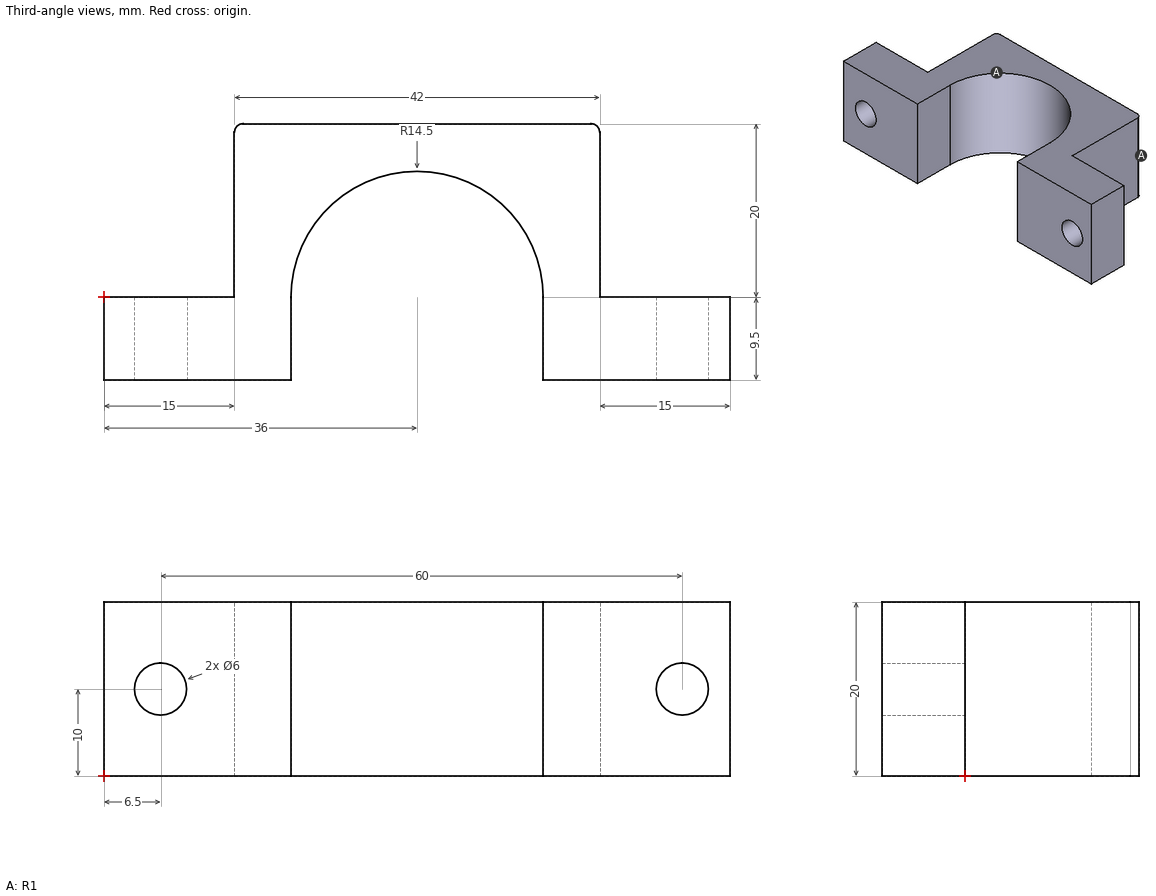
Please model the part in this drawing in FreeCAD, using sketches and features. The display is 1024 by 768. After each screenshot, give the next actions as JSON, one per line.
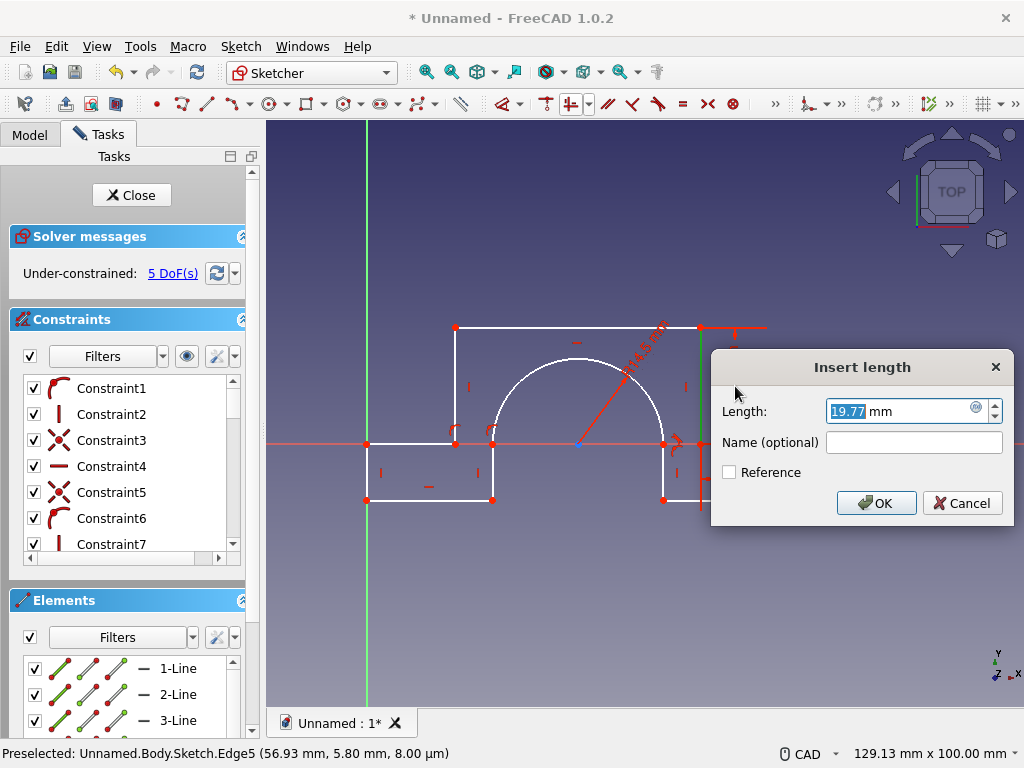
{"action": "type", "text": "20"}
{"action": "key", "text": "Return"}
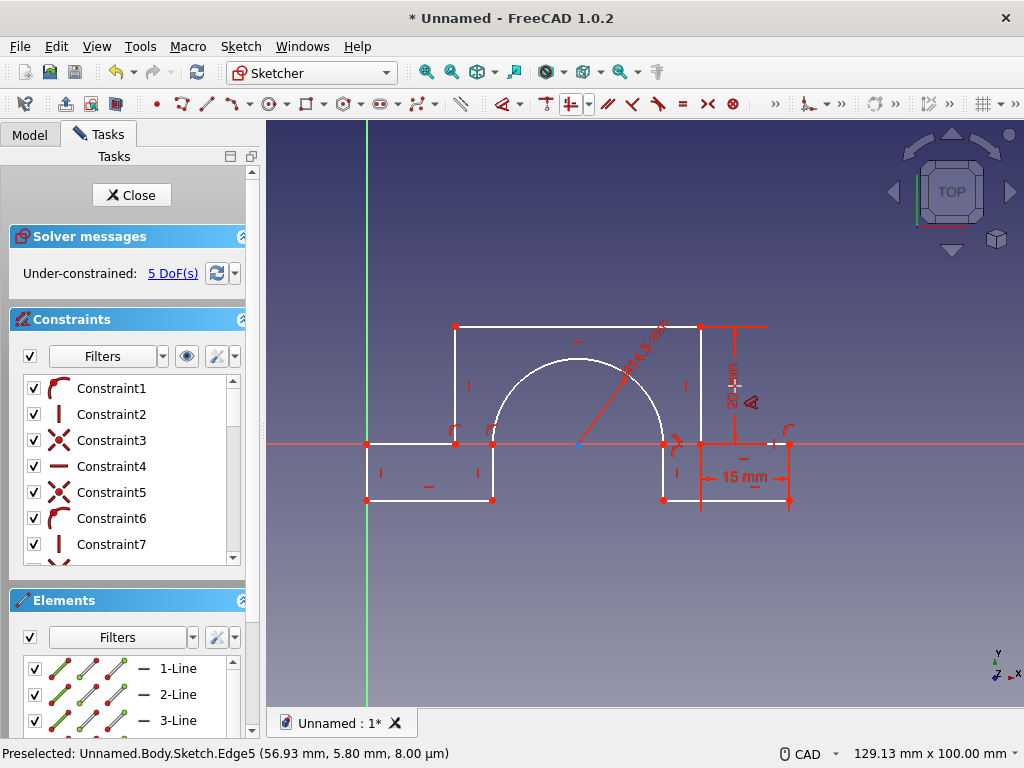
{"action": "left_click", "coordinate": [627, 327]}
{"action": "left_click", "coordinate": [578, 293]}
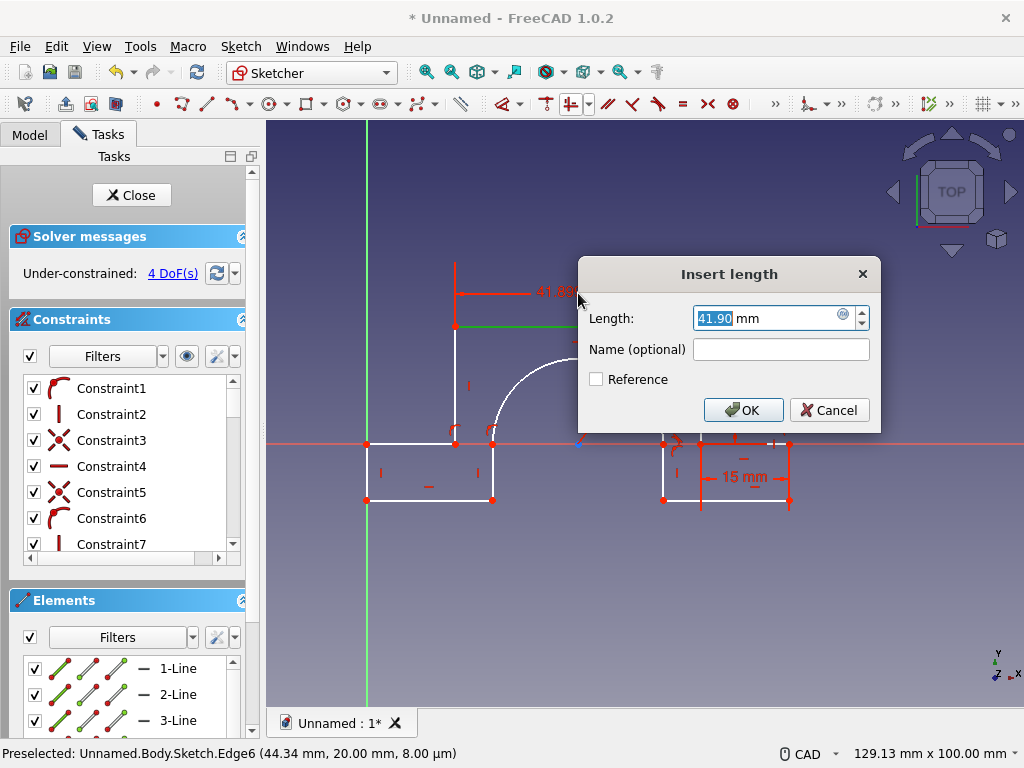
{"action": "type", "text": "42"}
{"action": "key", "text": "Return"}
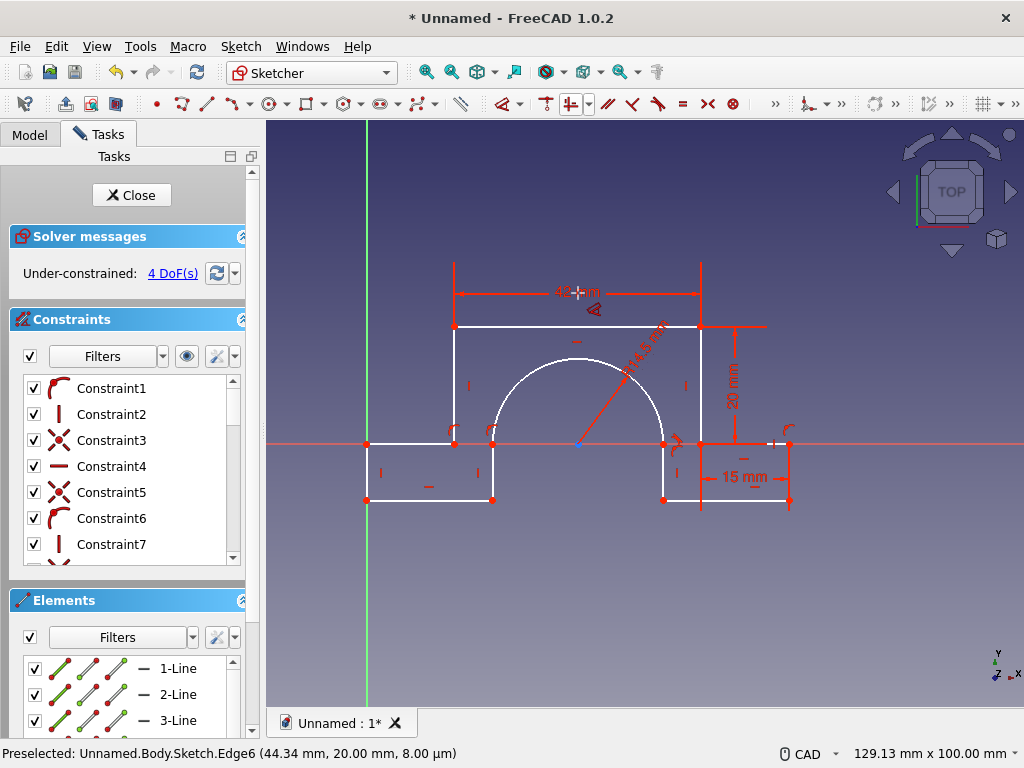
{"action": "left_click", "coordinate": [428, 444]}
{"action": "left_click", "coordinate": [411, 478]}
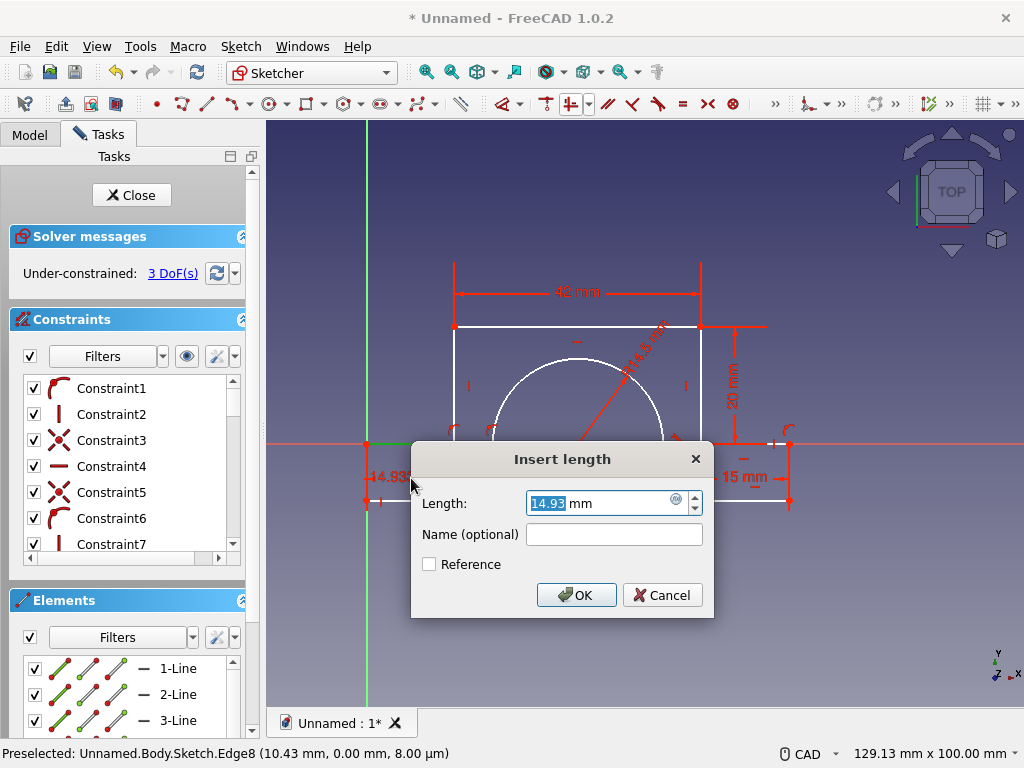
{"action": "type", "text": "15"}
{"action": "key", "text": "Return"}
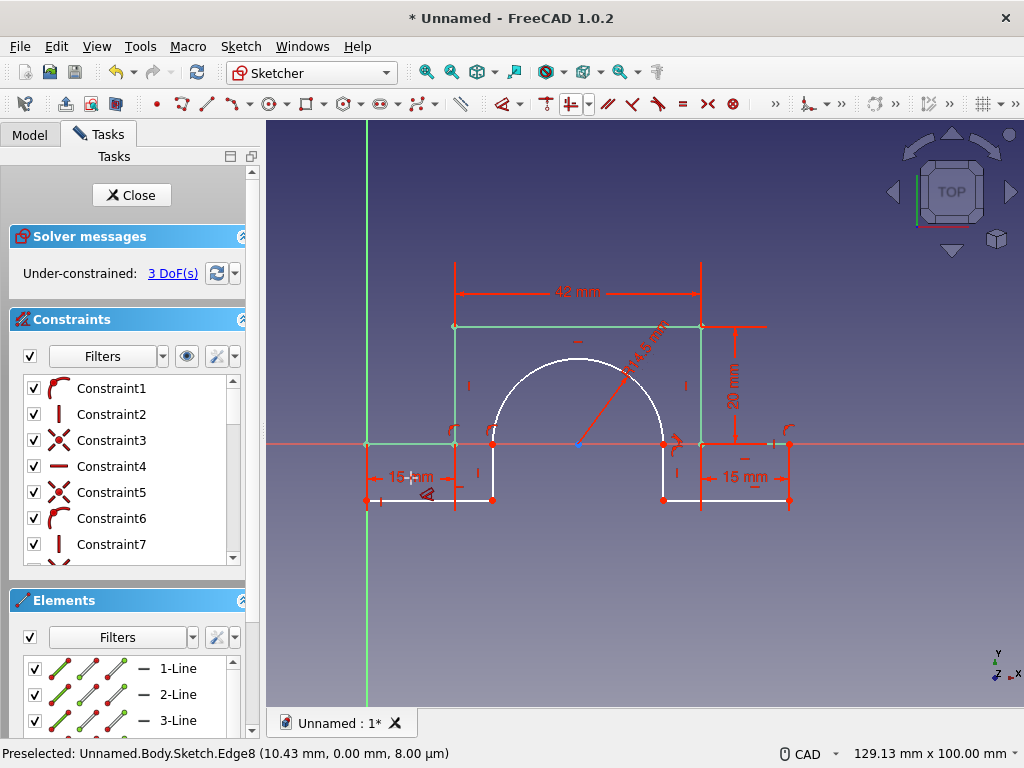
{"action": "left_click", "coordinate": [663, 461]}
{"action": "left_click", "coordinate": [629, 473]}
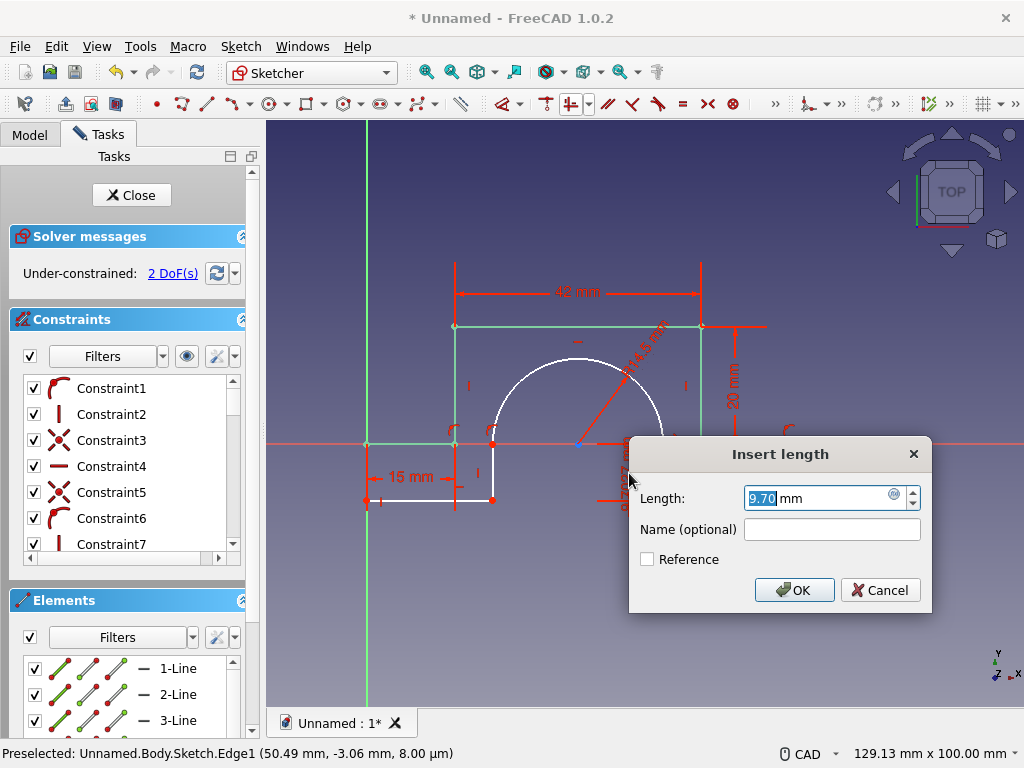
{"action": "type", "text": "9.5"}
{"action": "key", "text": "Return"}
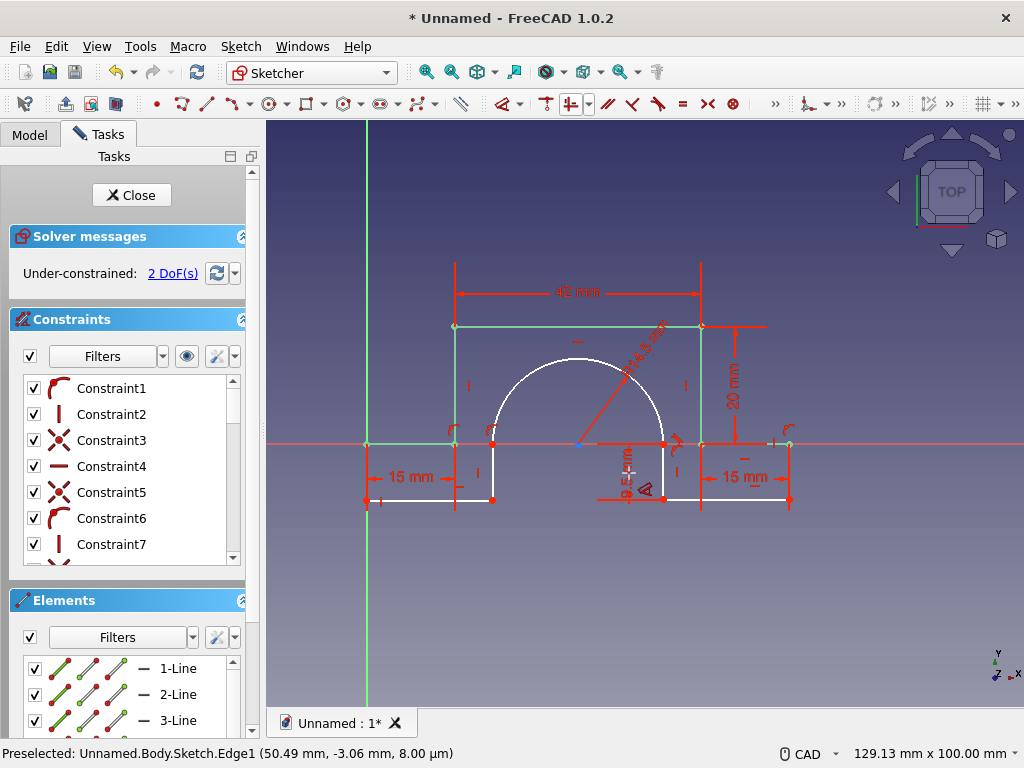
{"action": "left_click", "coordinate": [367, 461]}
{"action": "left_click", "coordinate": [333, 473]}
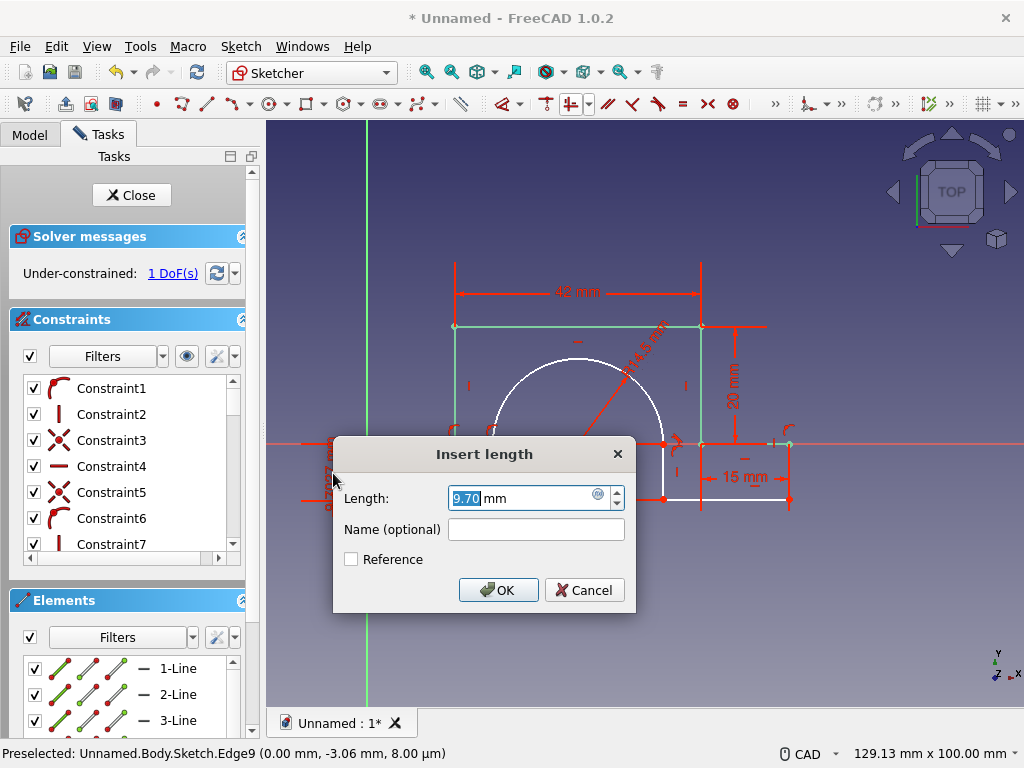
{"action": "type", "text": "9.5"}
{"action": "key", "text": "Return"}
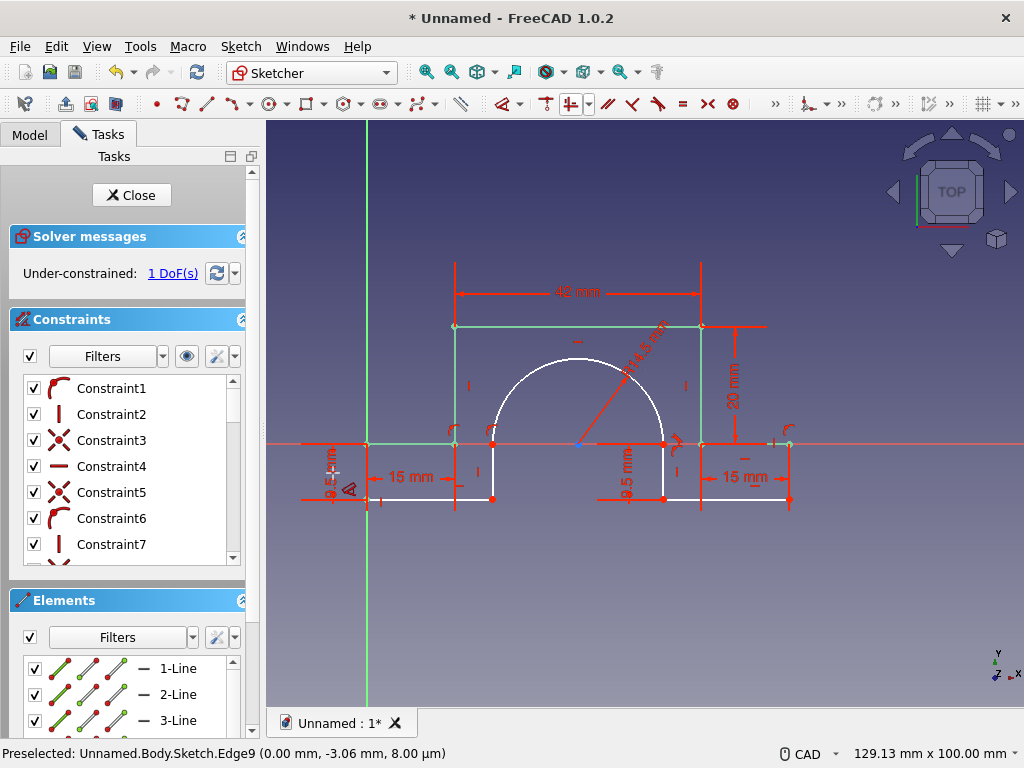
{"action": "left_click", "coordinate": [578, 444]}
{"action": "left_click", "coordinate": [521, 478]}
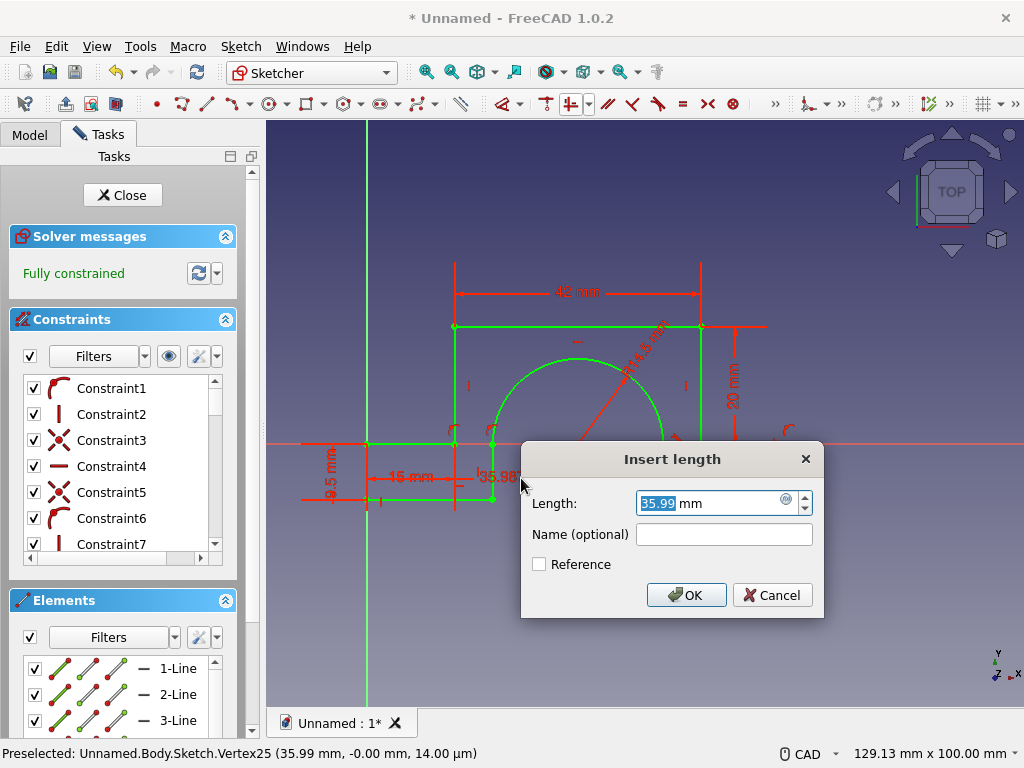
{"action": "type", "text": "36"}
{"action": "key", "text": "Return"}
{"action": "key", "text": "Escape"}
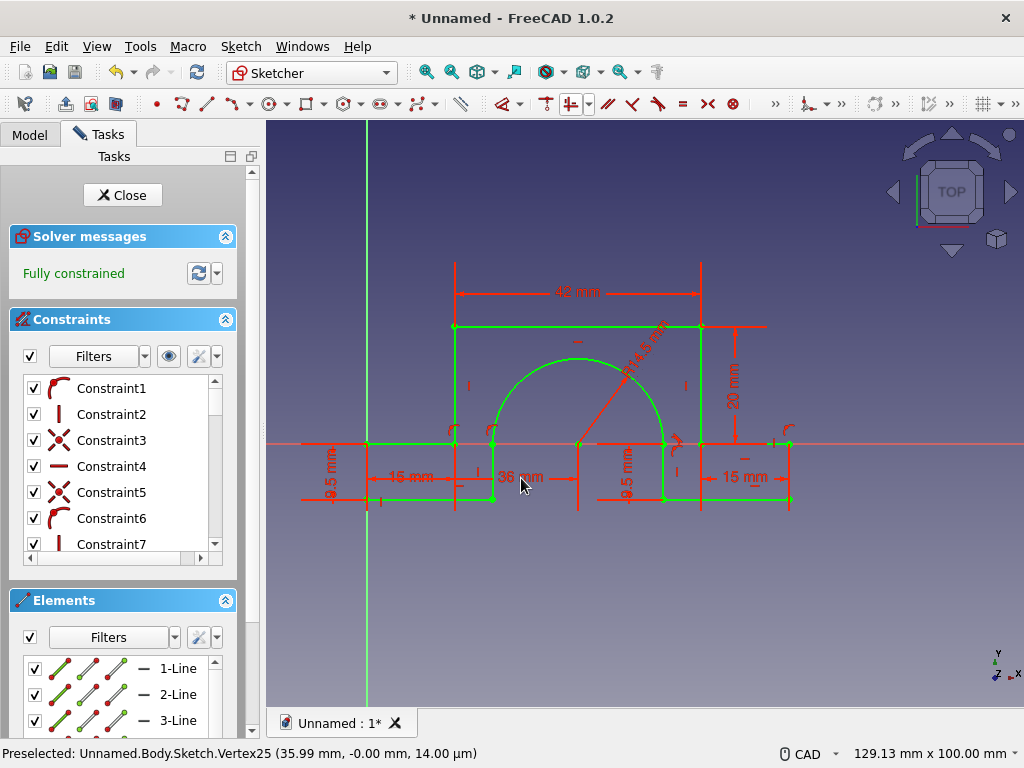
{"action": "left_click", "coordinate": [123, 195]}